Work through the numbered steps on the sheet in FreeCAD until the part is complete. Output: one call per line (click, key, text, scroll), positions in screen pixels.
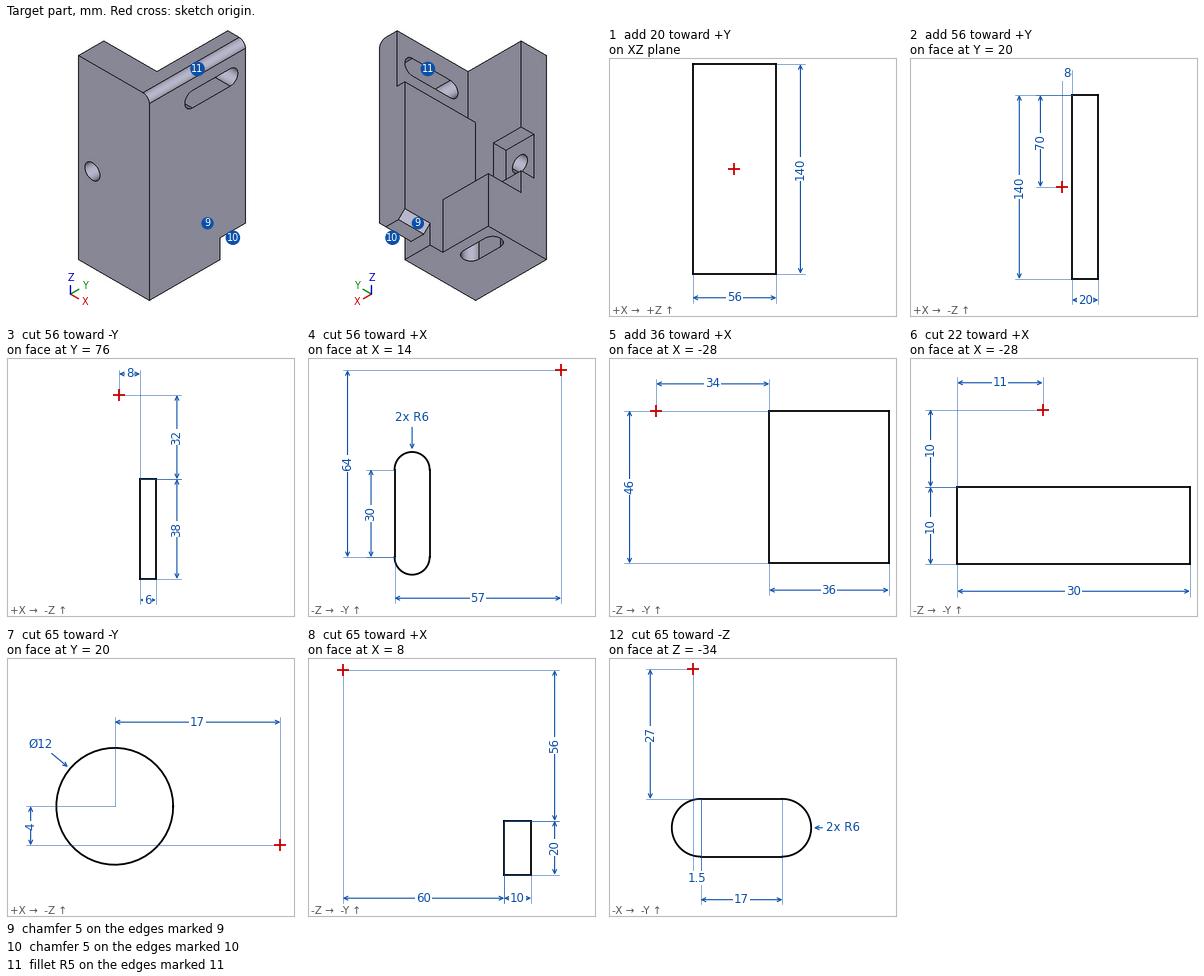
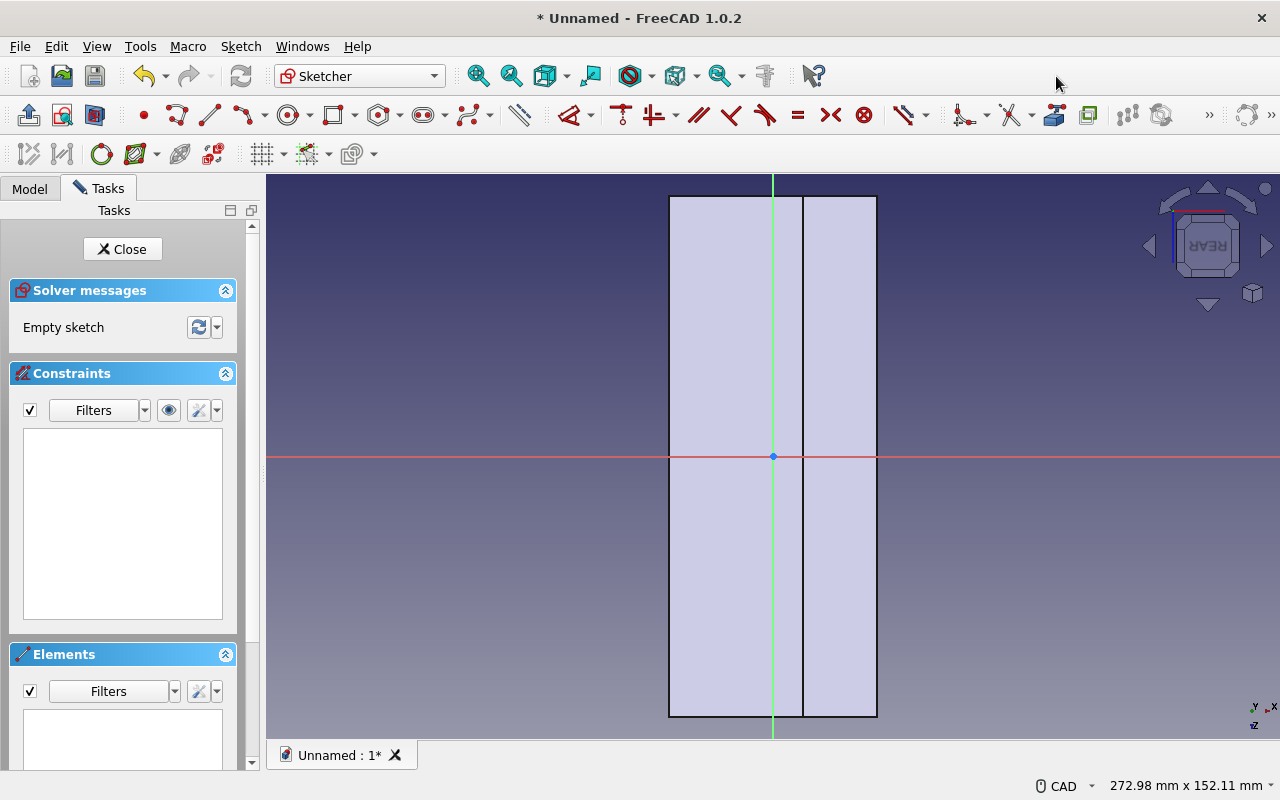
scroll(294, 202, down, 1)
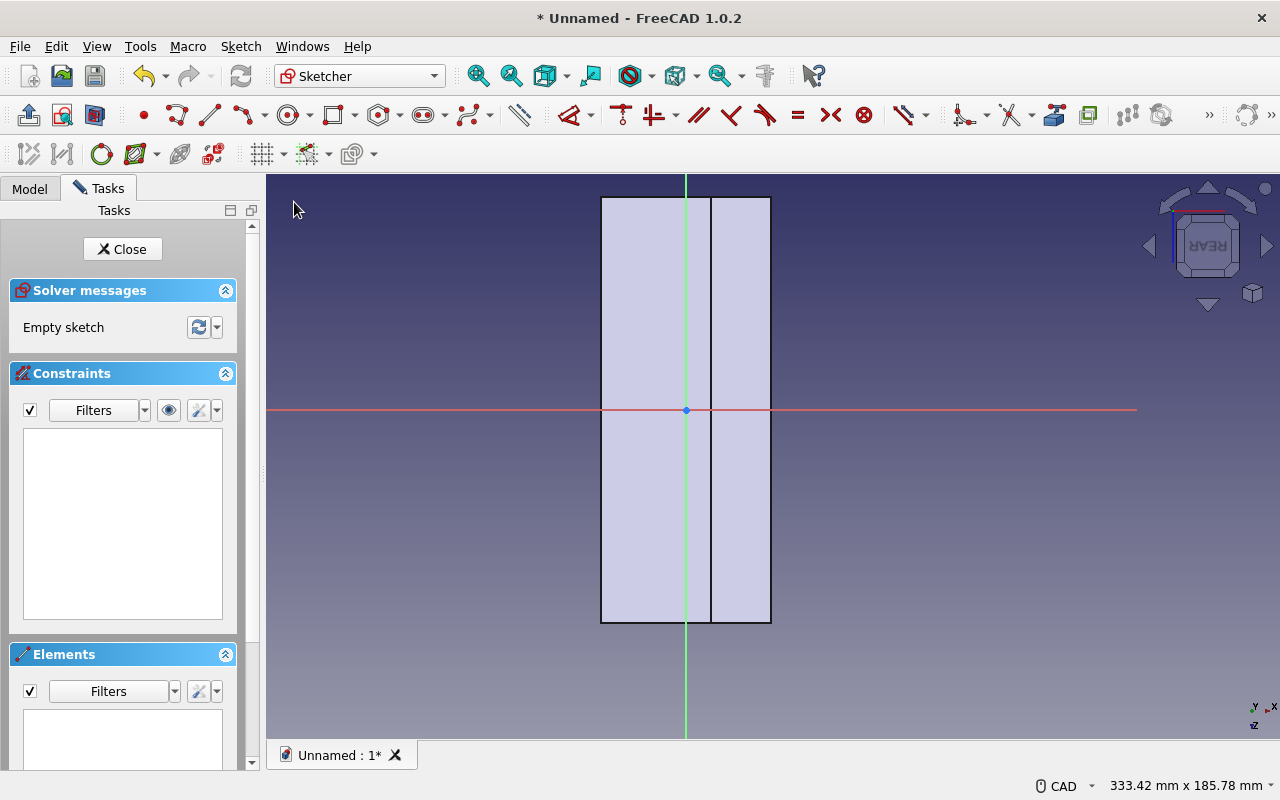
scroll(711, 590, up, 3)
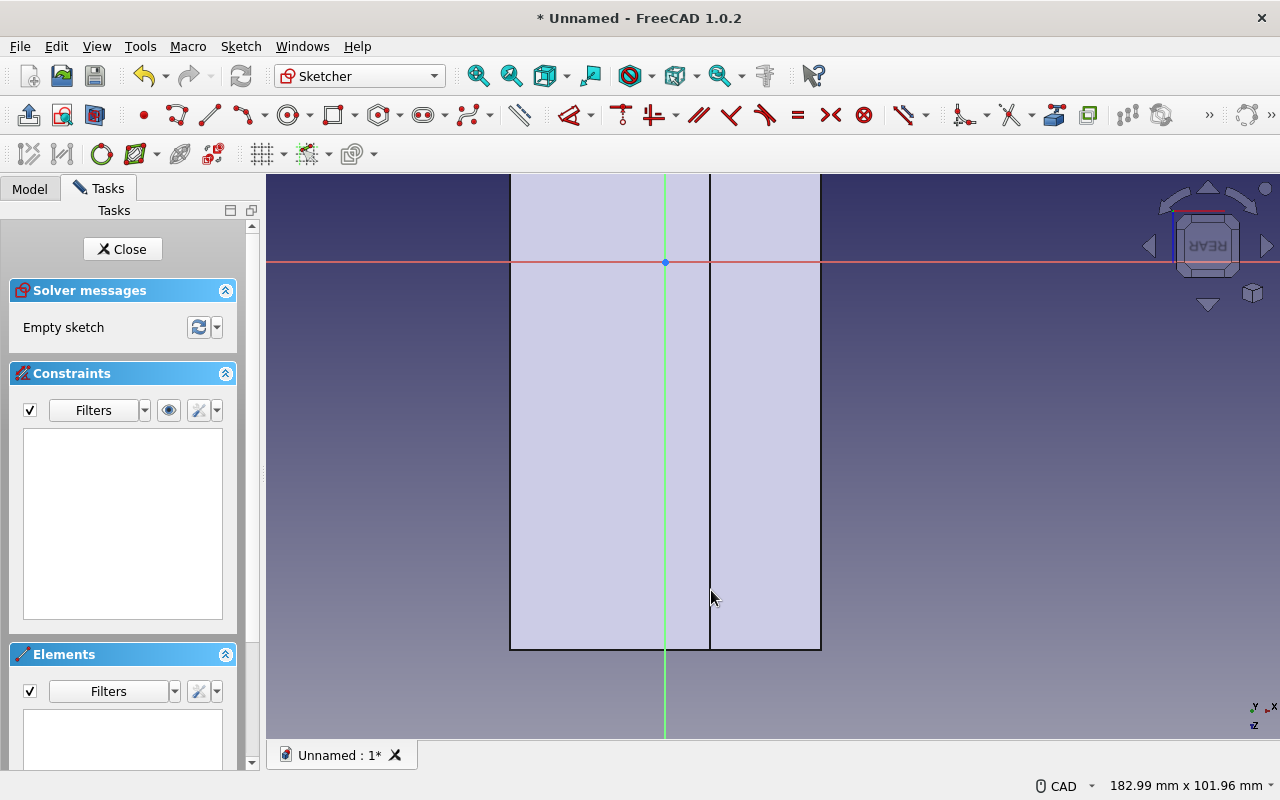
click(332, 116)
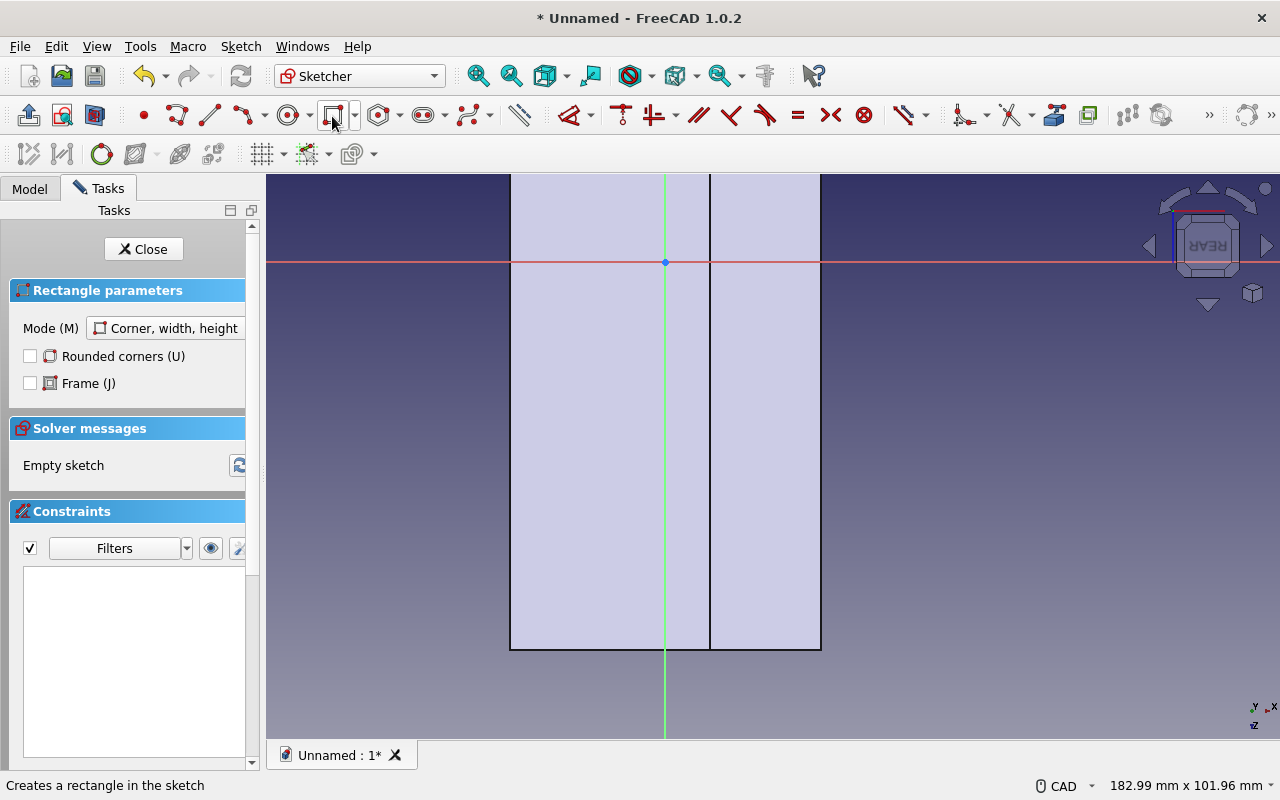
click(710, 439)
click(743, 650)
key(Escape)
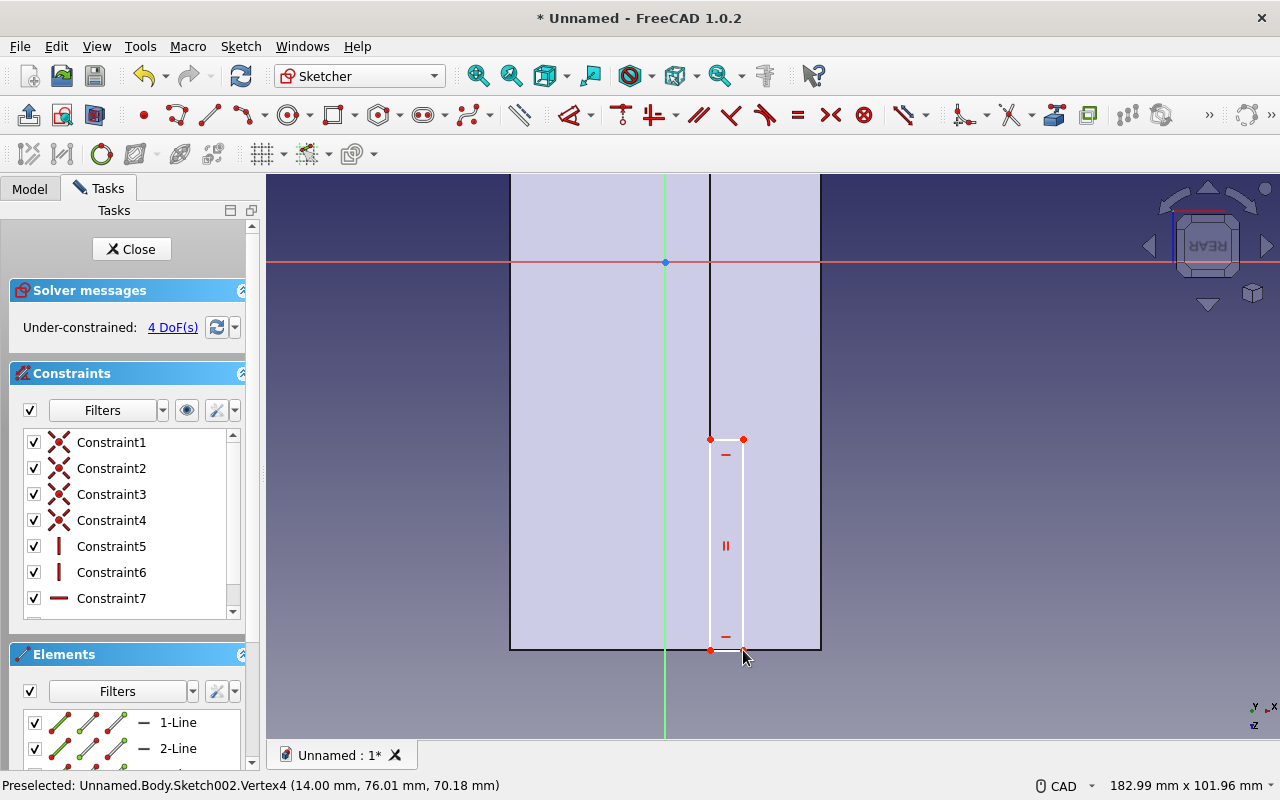
click(568, 116)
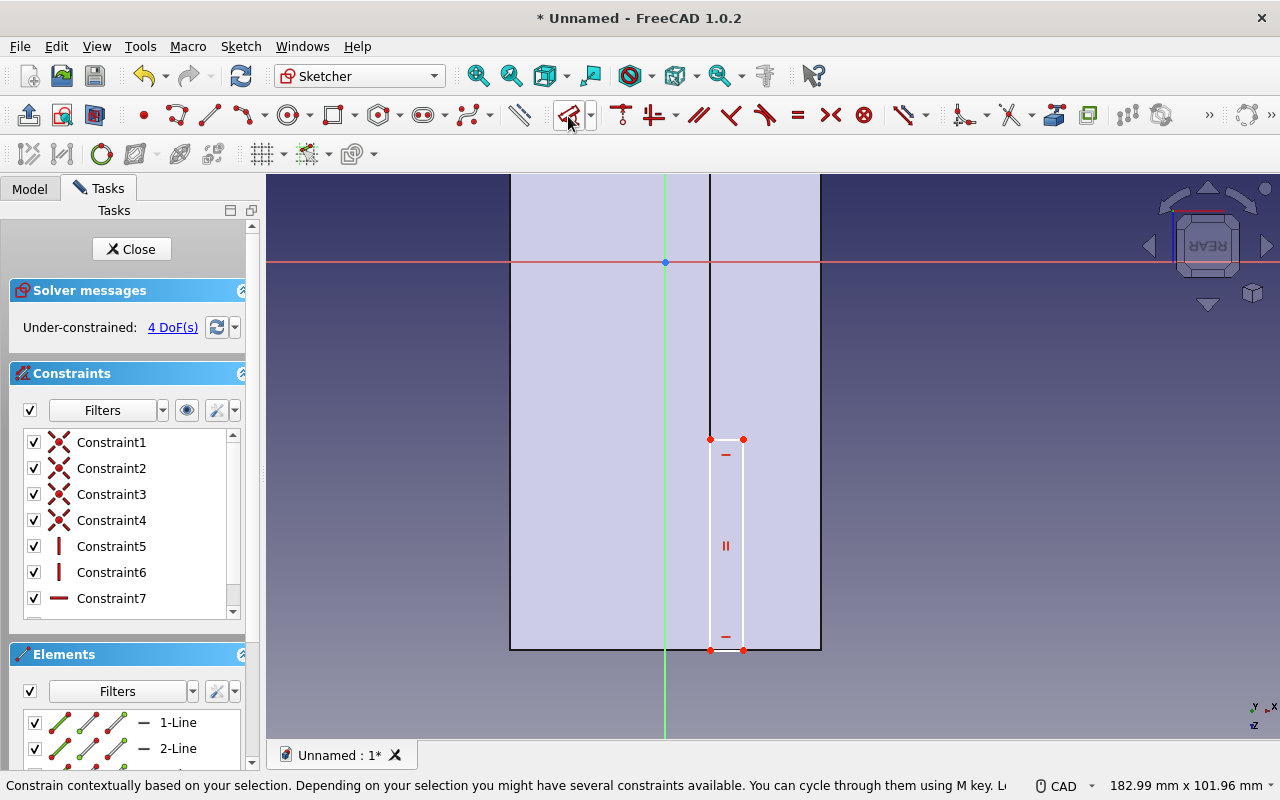
scroll(720, 651, up, 2)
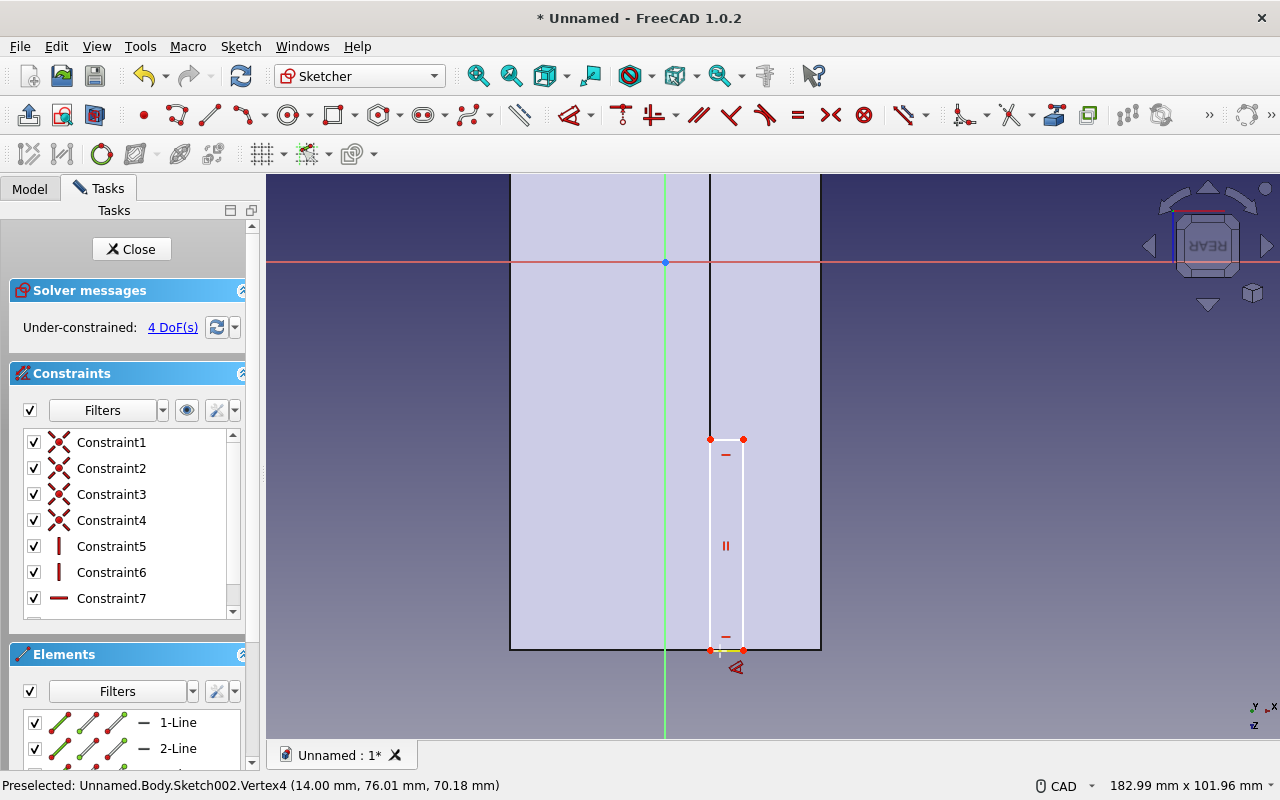
click(720, 651)
click(729, 685)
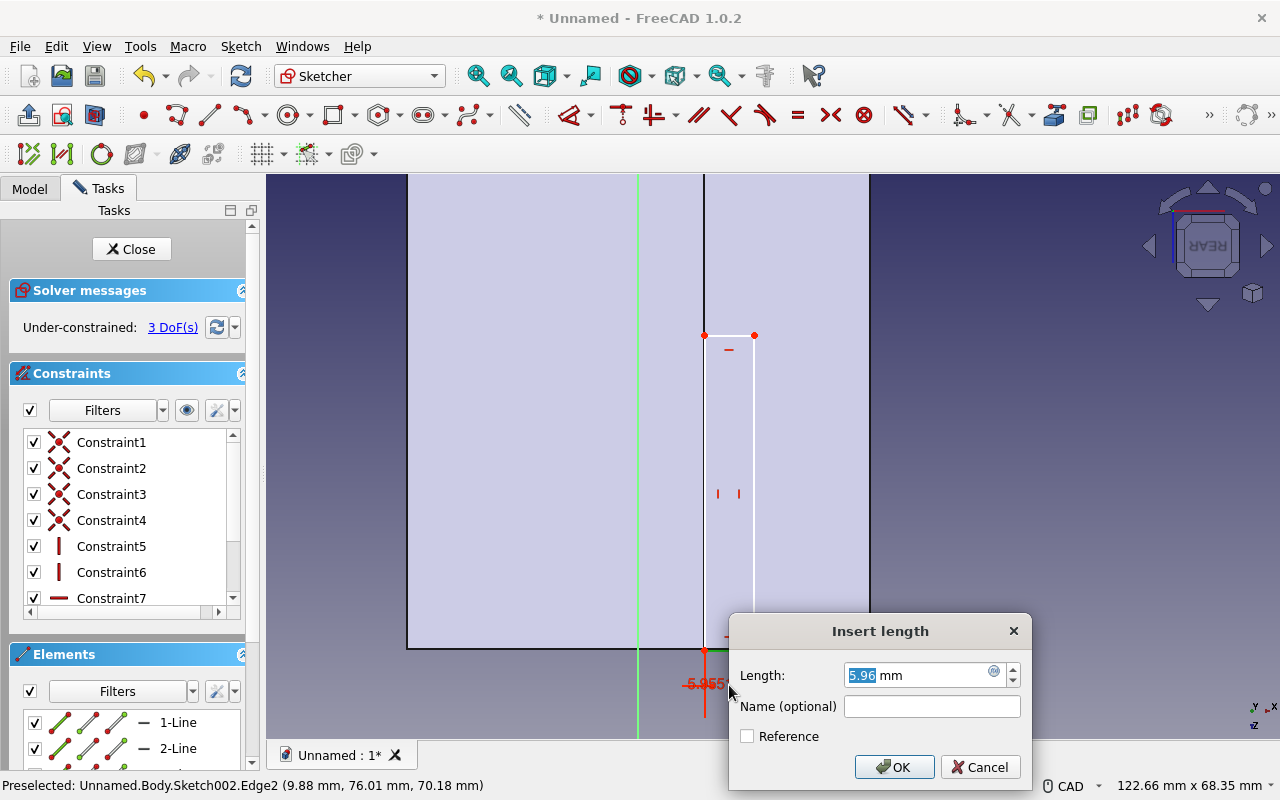
text(6)
key(Return)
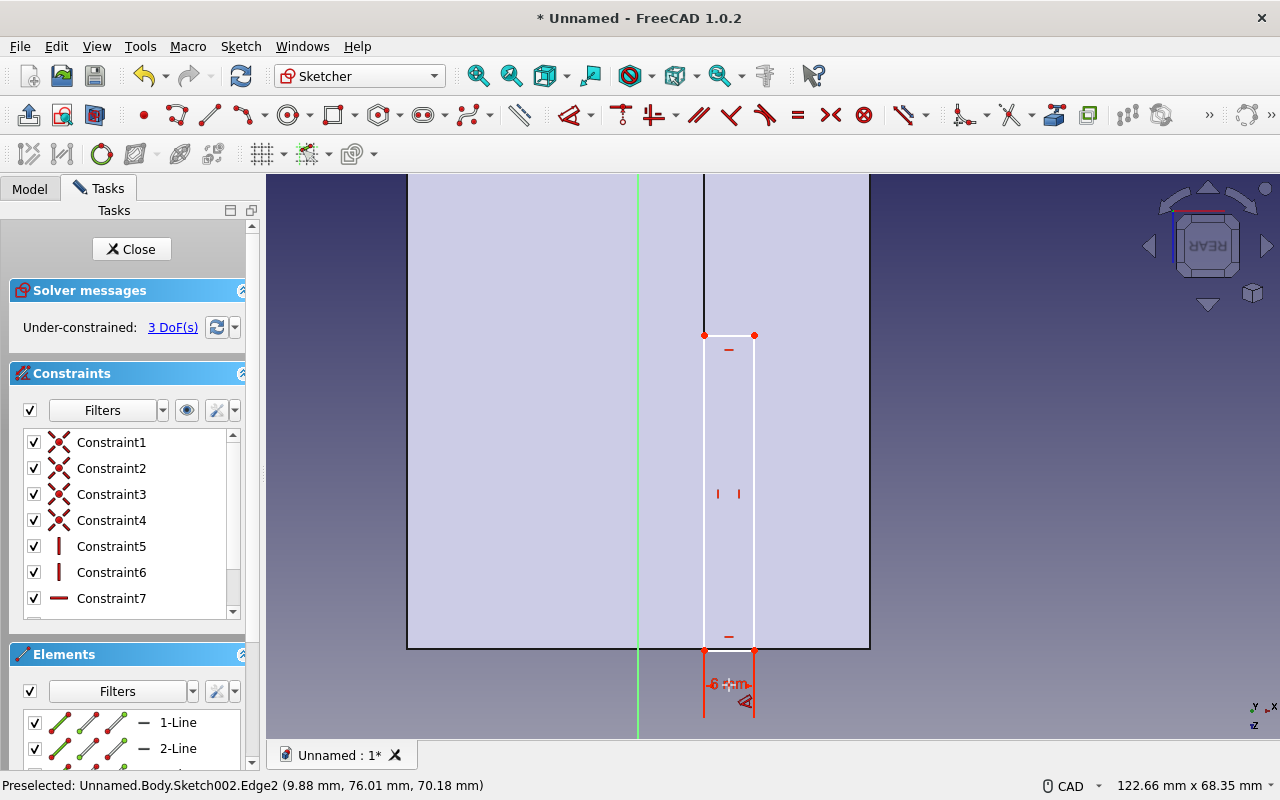
click(704, 430)
click(738, 493)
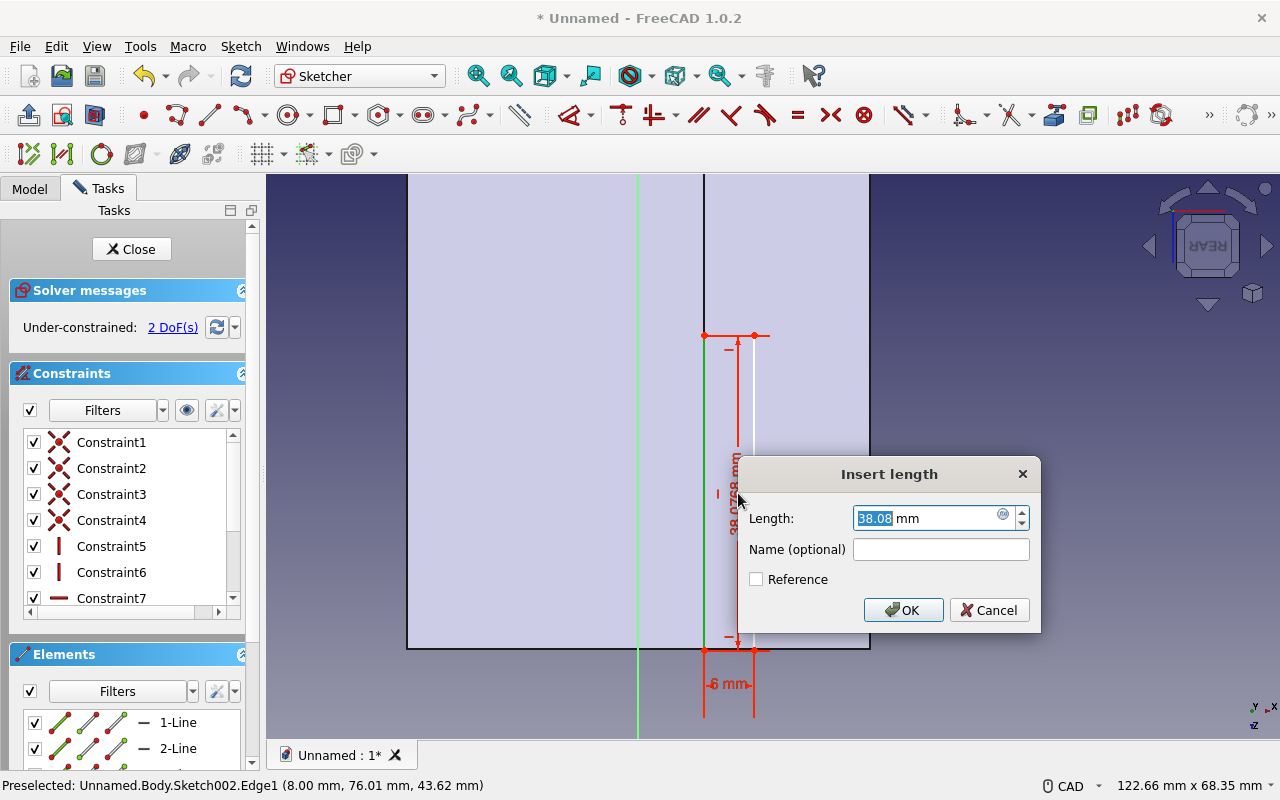
text(38)
key(Return)